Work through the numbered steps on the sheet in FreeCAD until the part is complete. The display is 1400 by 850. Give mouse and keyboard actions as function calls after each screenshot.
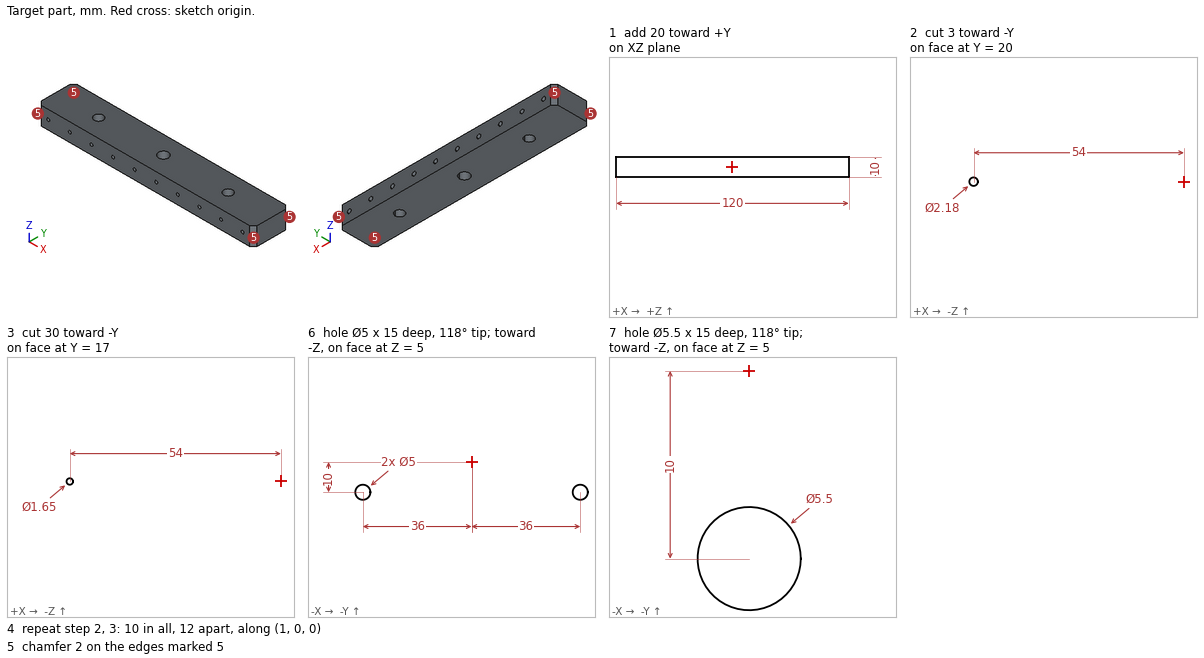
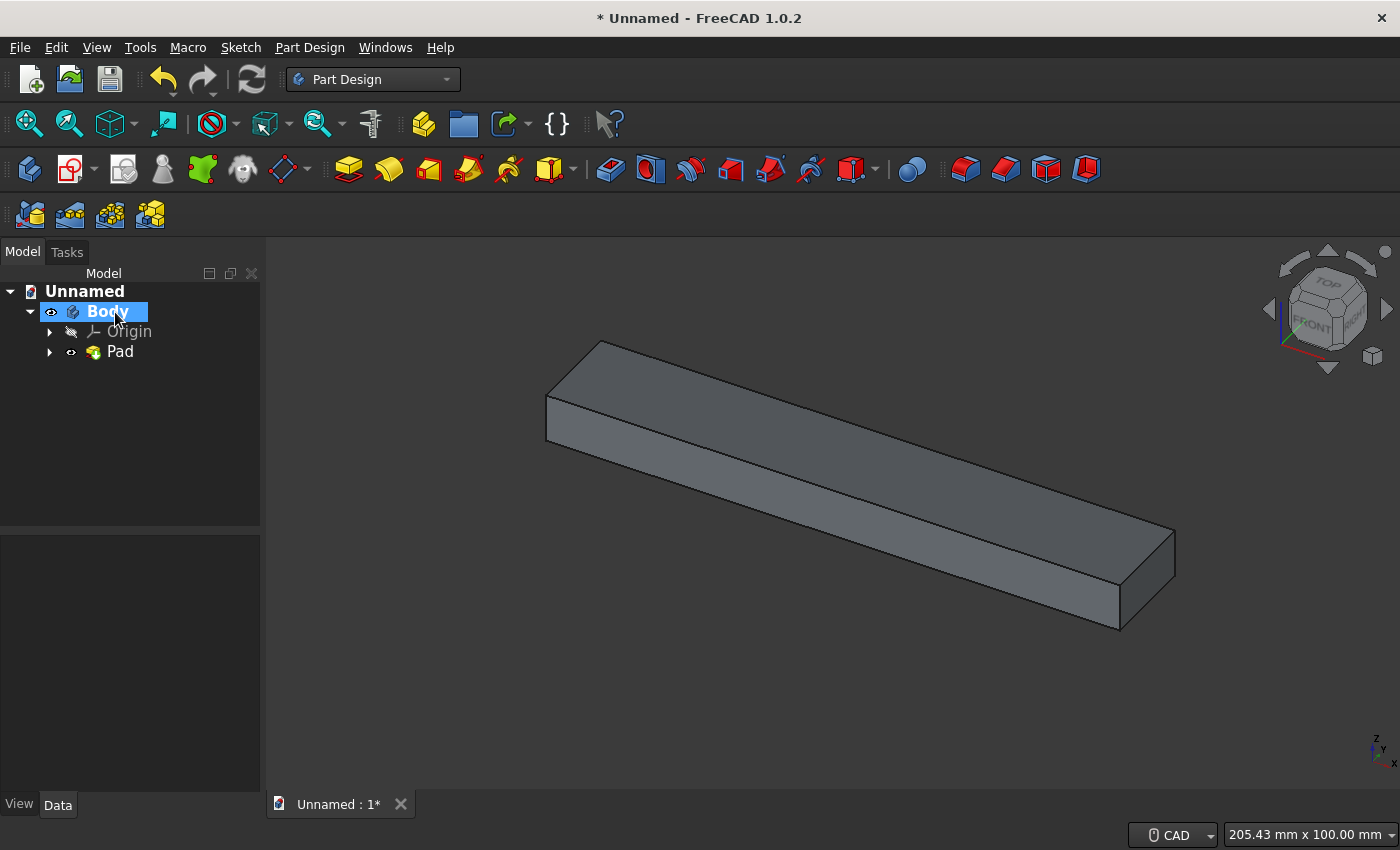
key(4)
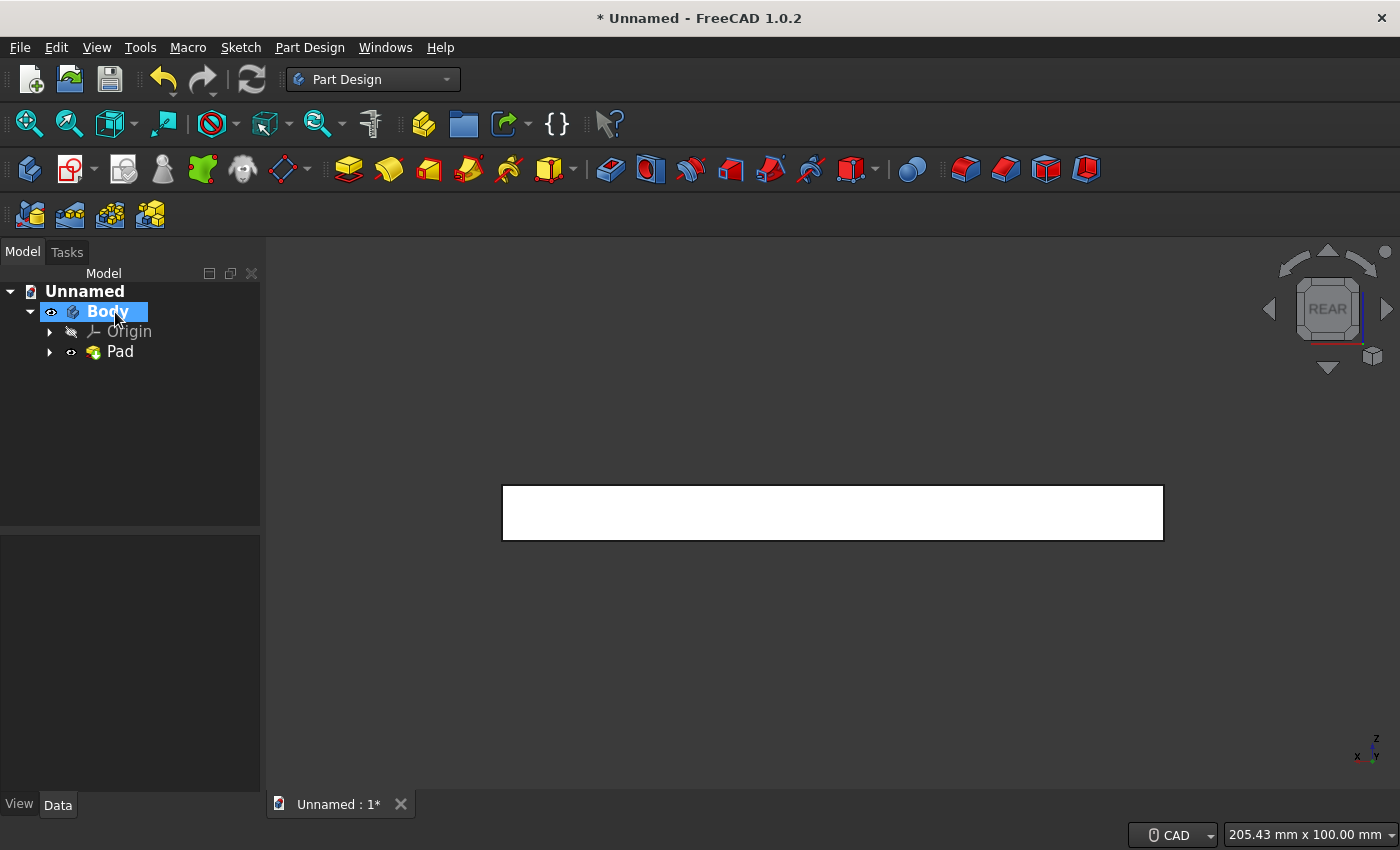
click(549, 512)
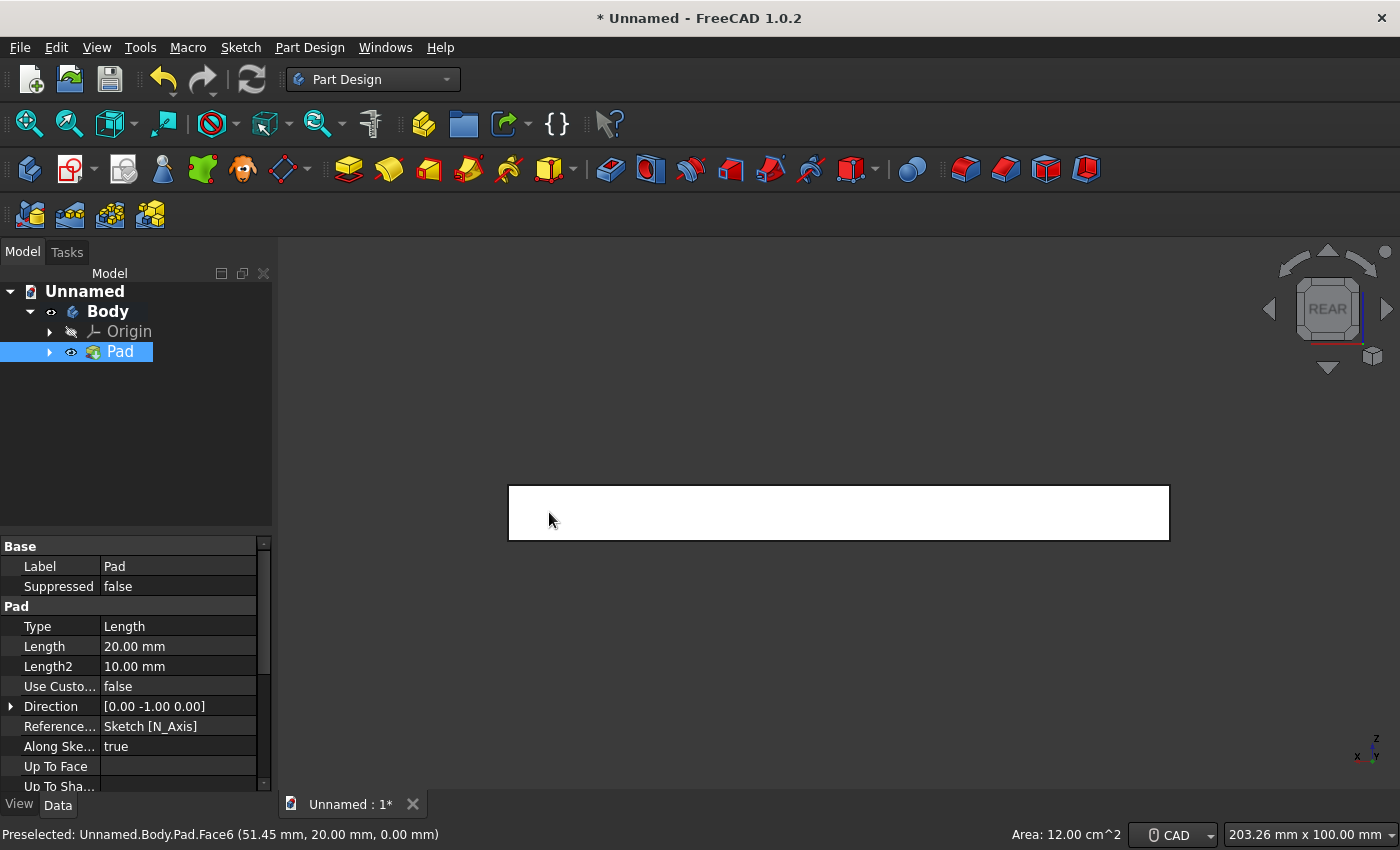
click(70, 170)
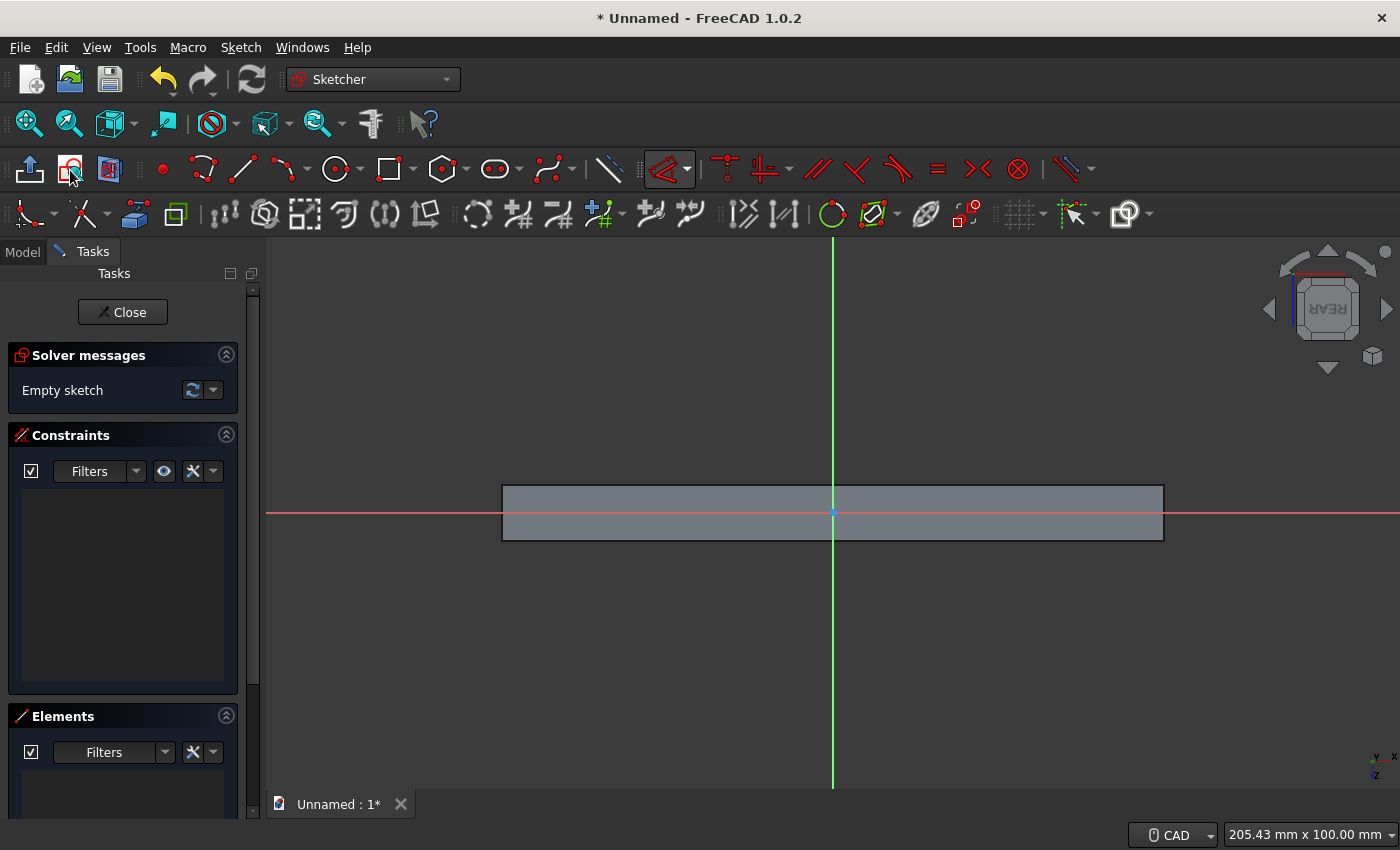
scroll(523, 513, up, 15)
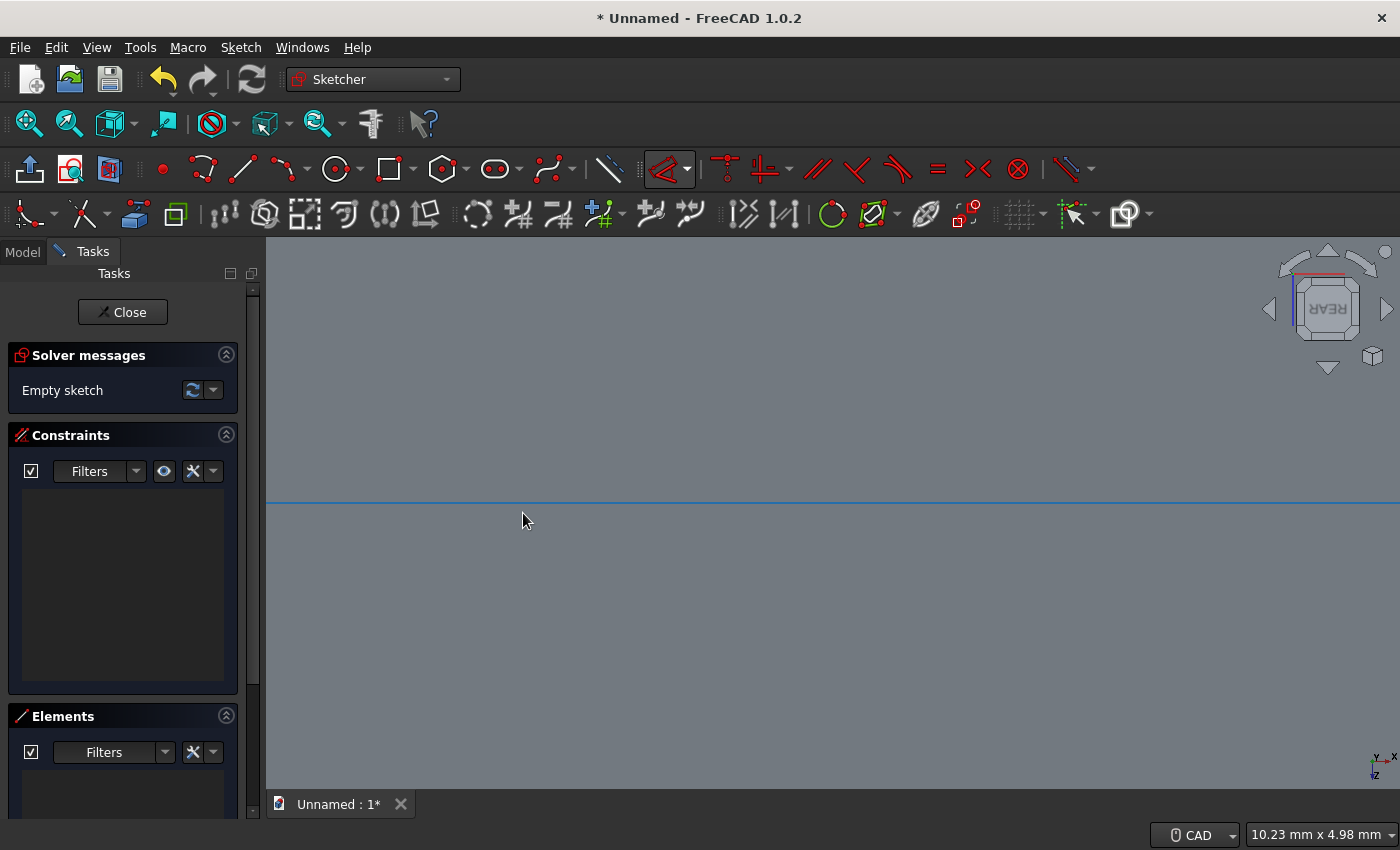
scroll(745, 484, up, 2)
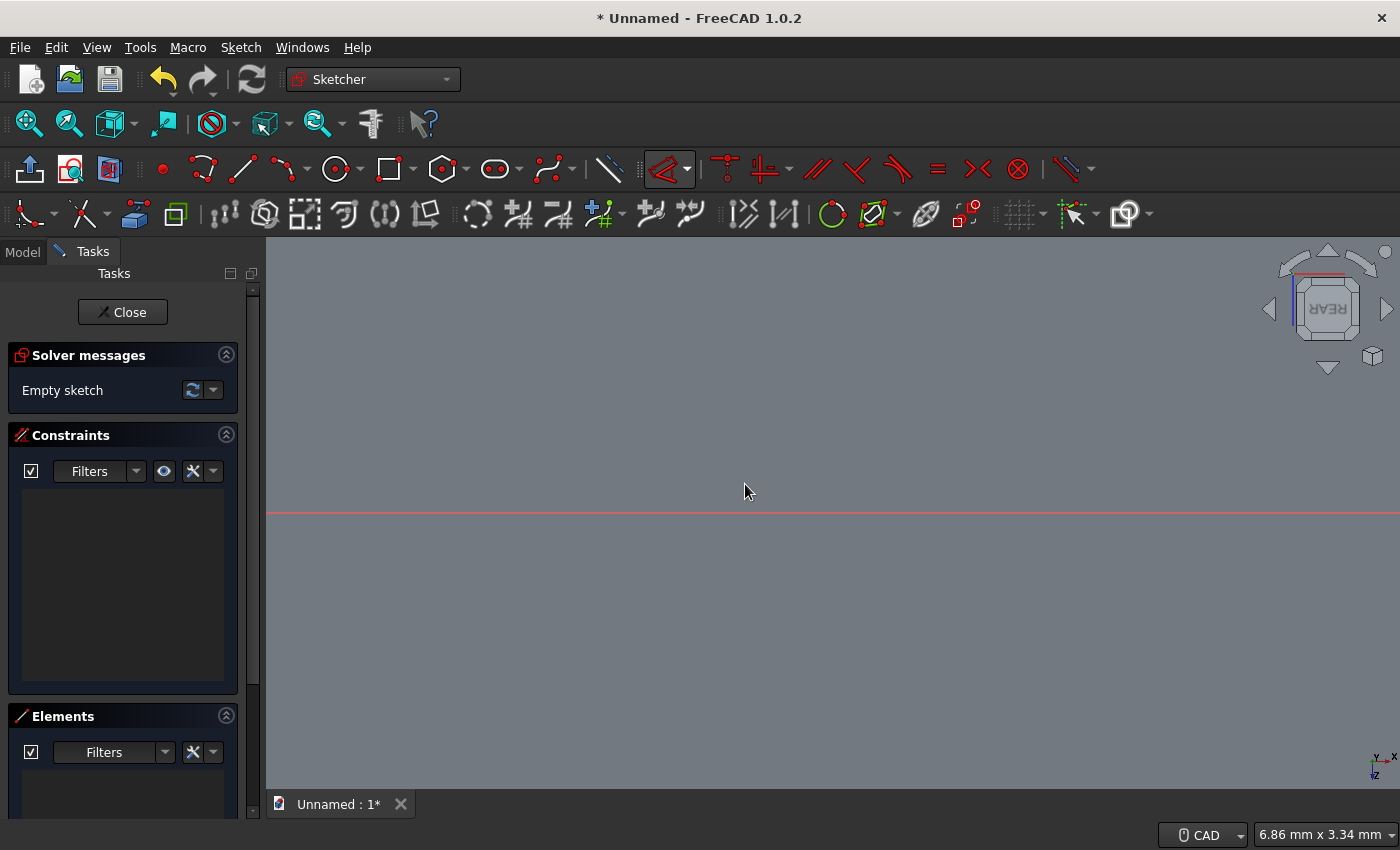
click(336, 170)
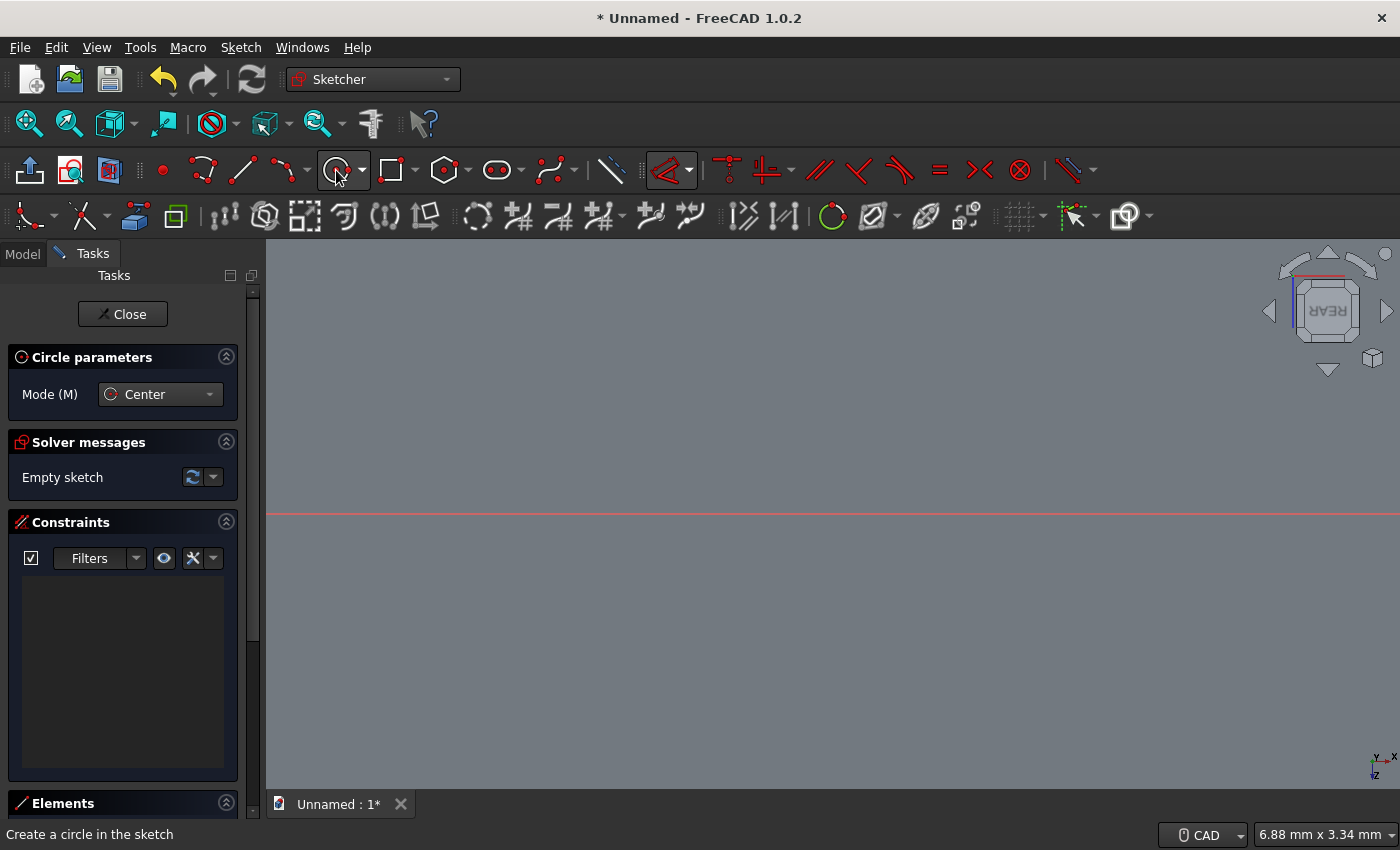
click(765, 514)
click(892, 387)
key(Escape)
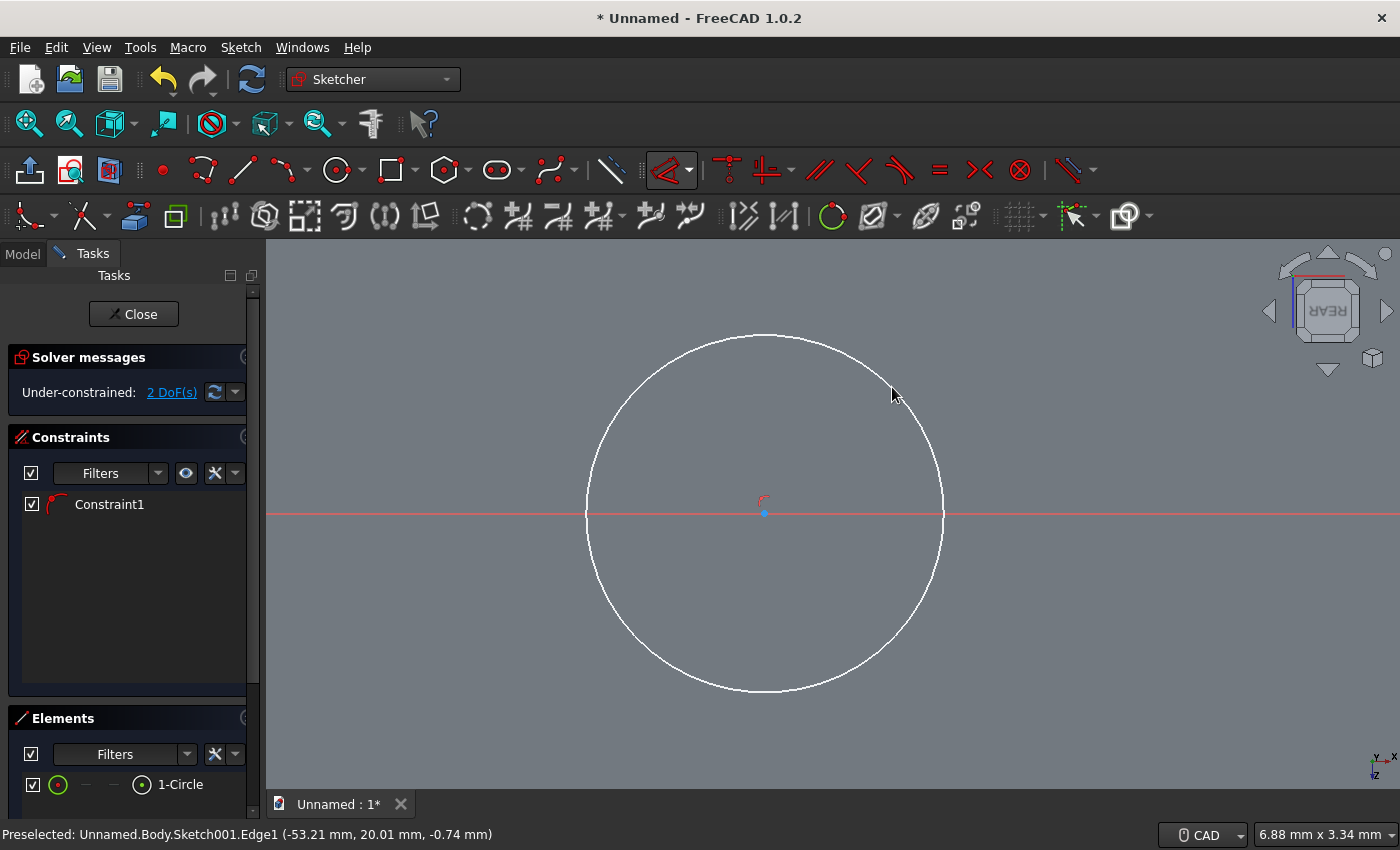
click(891, 387)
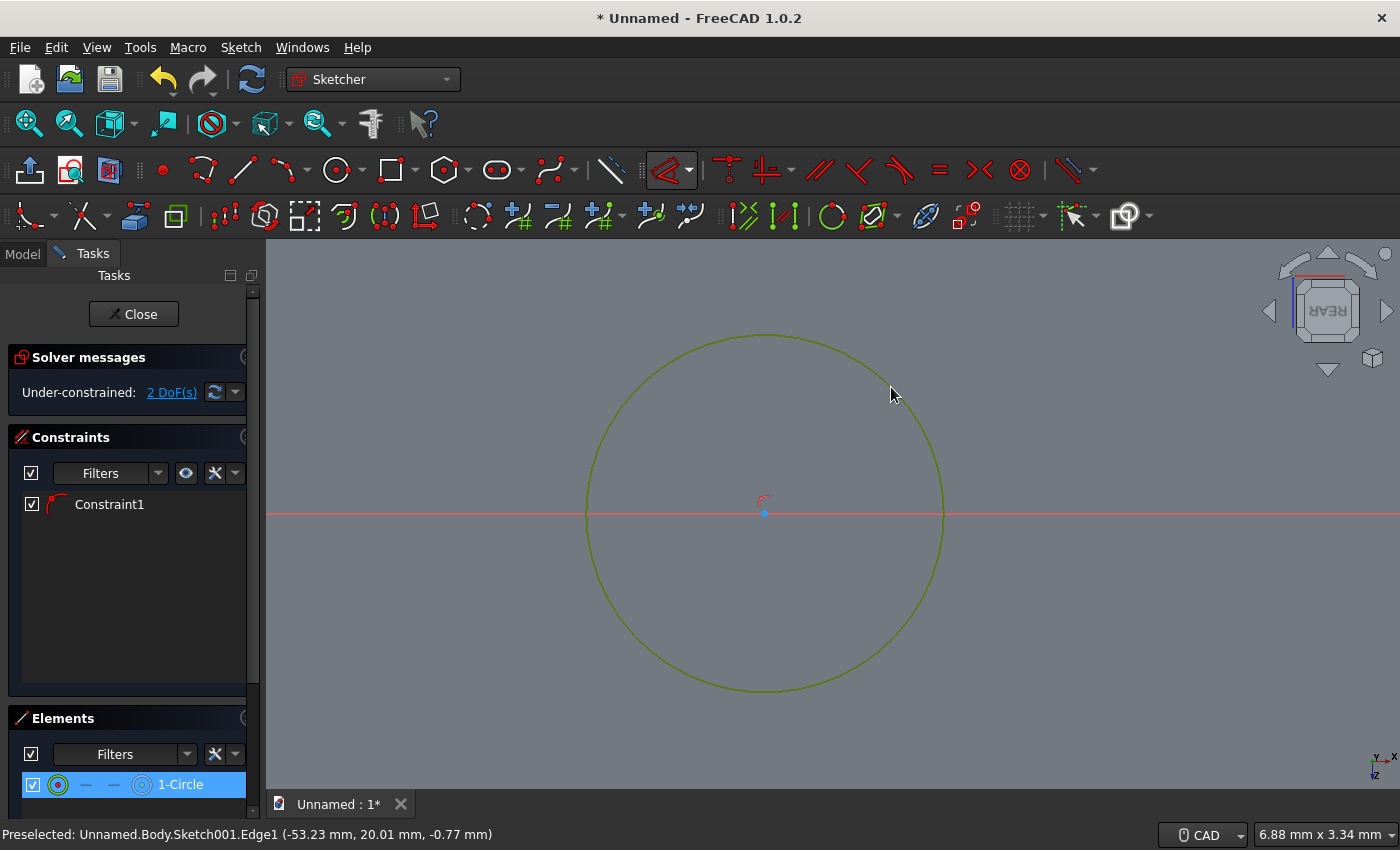
key(k)
key(o)